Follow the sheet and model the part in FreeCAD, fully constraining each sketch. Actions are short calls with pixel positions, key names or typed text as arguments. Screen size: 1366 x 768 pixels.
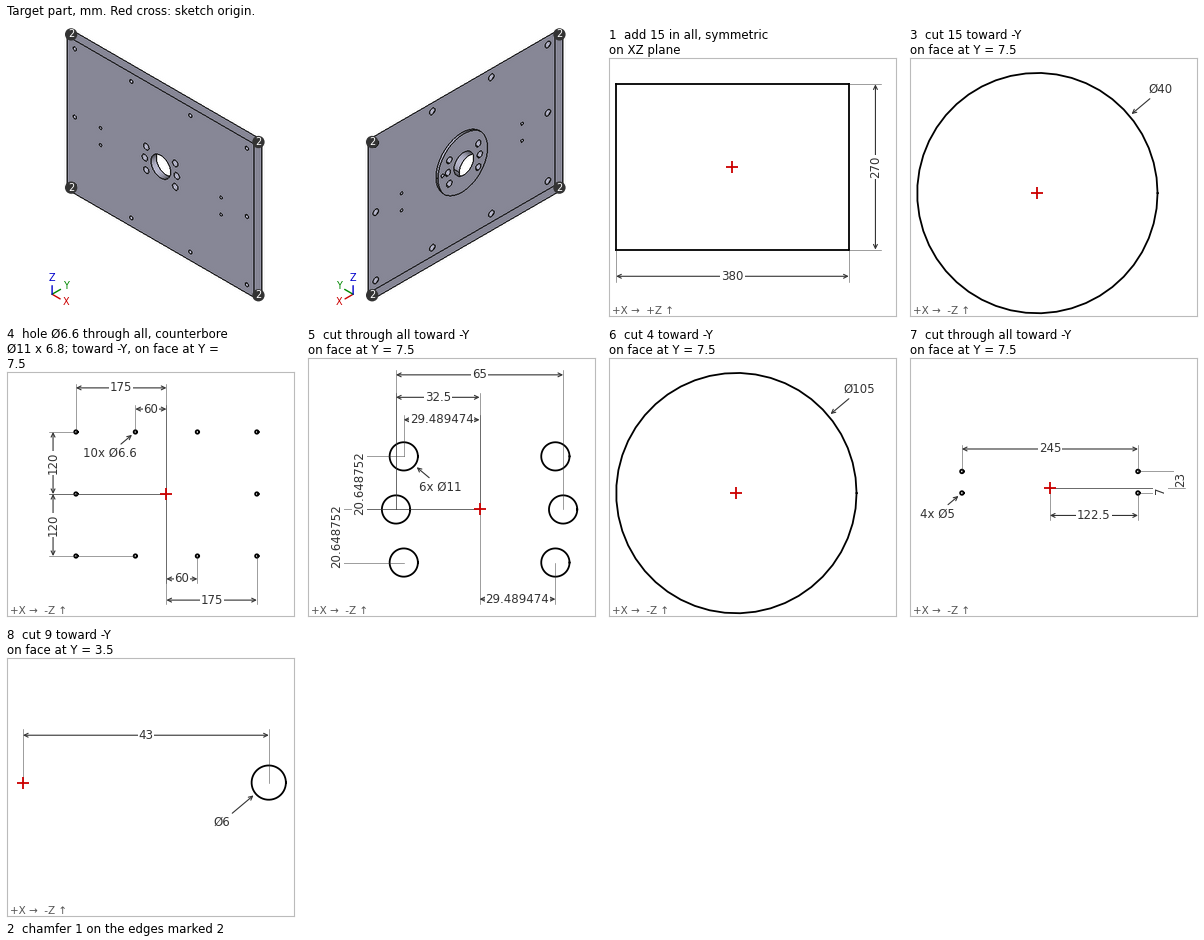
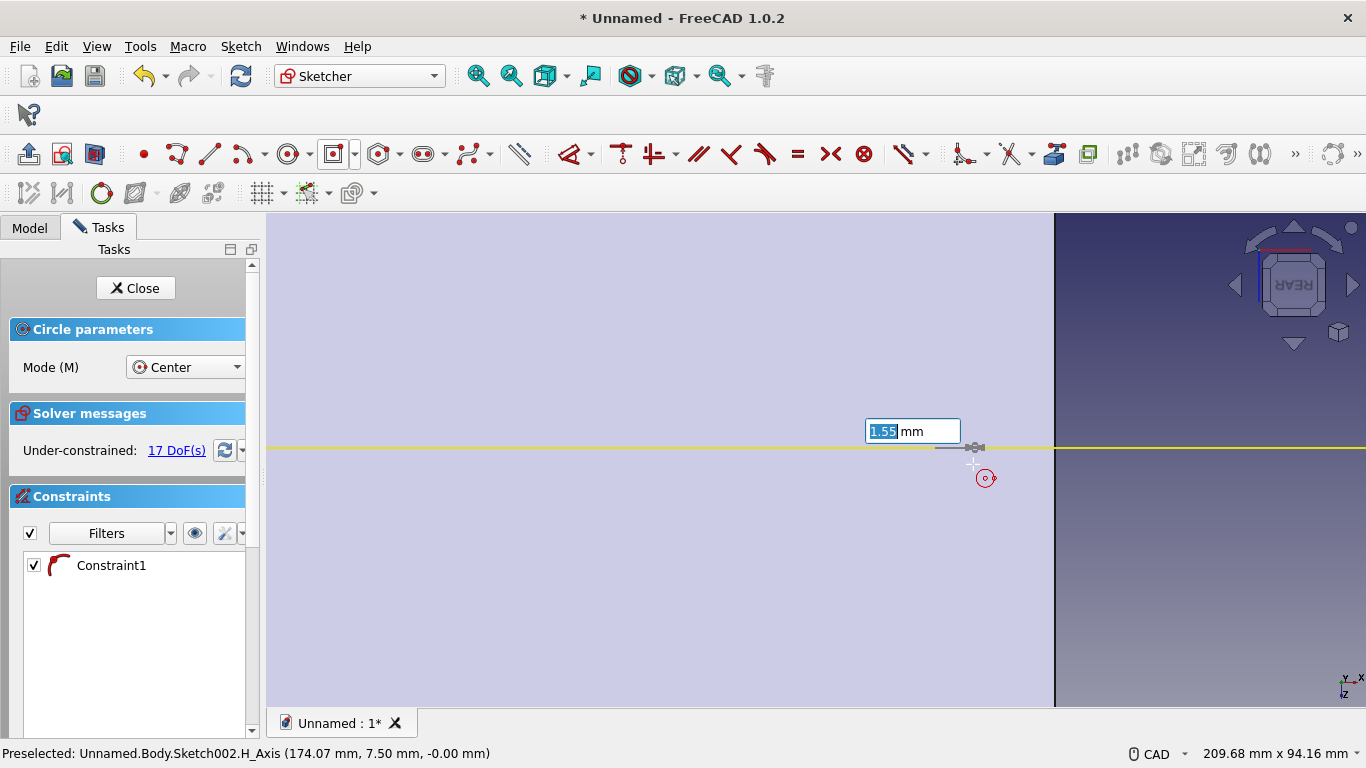
click(970, 464)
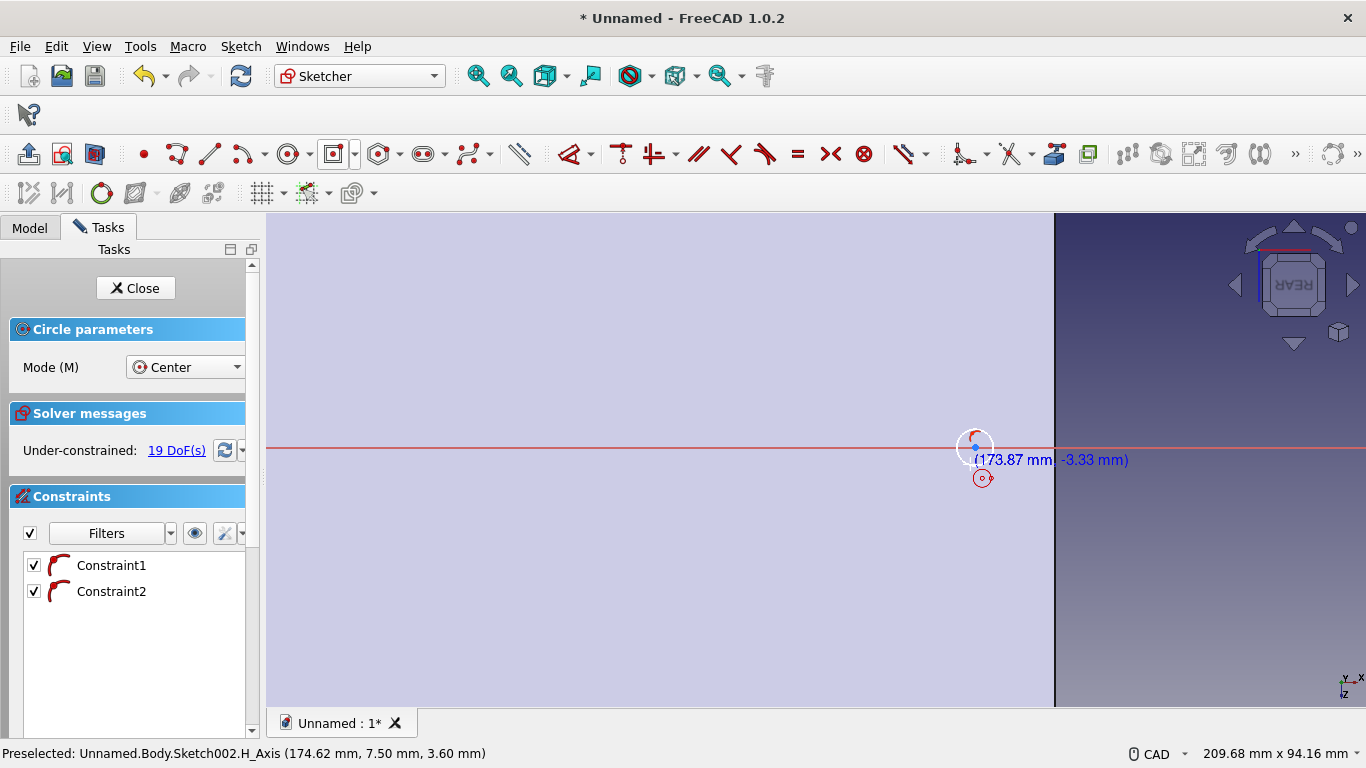
scroll(973, 464, down, 7)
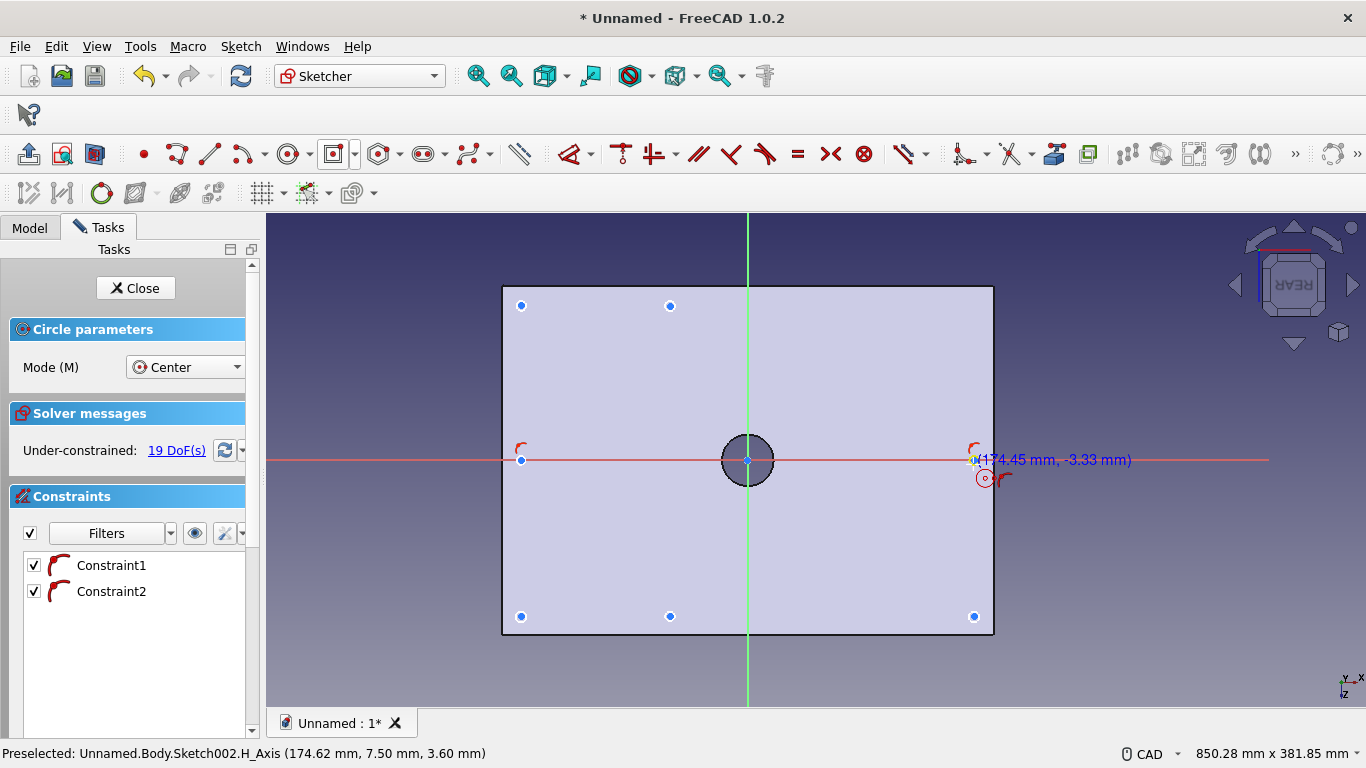
scroll(825, 616, up, 9)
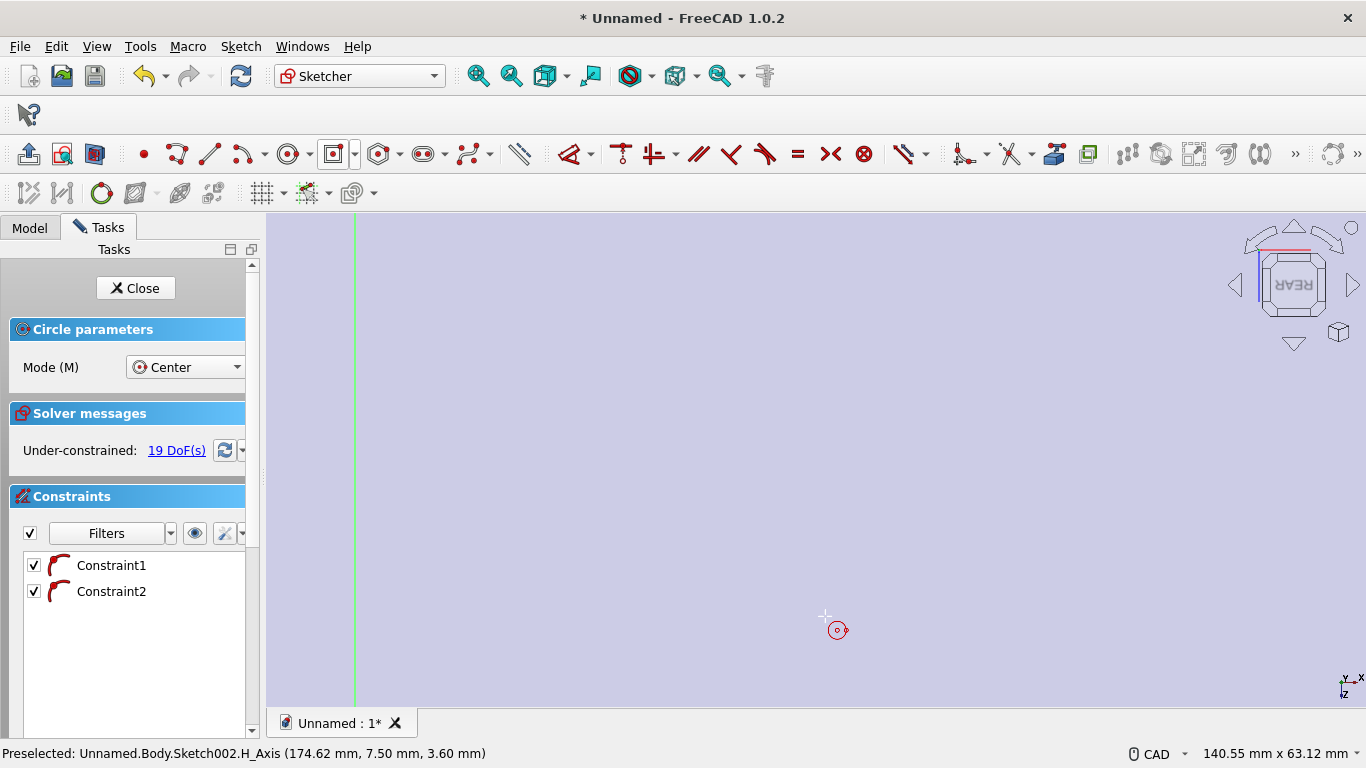
scroll(825, 616, down, 9)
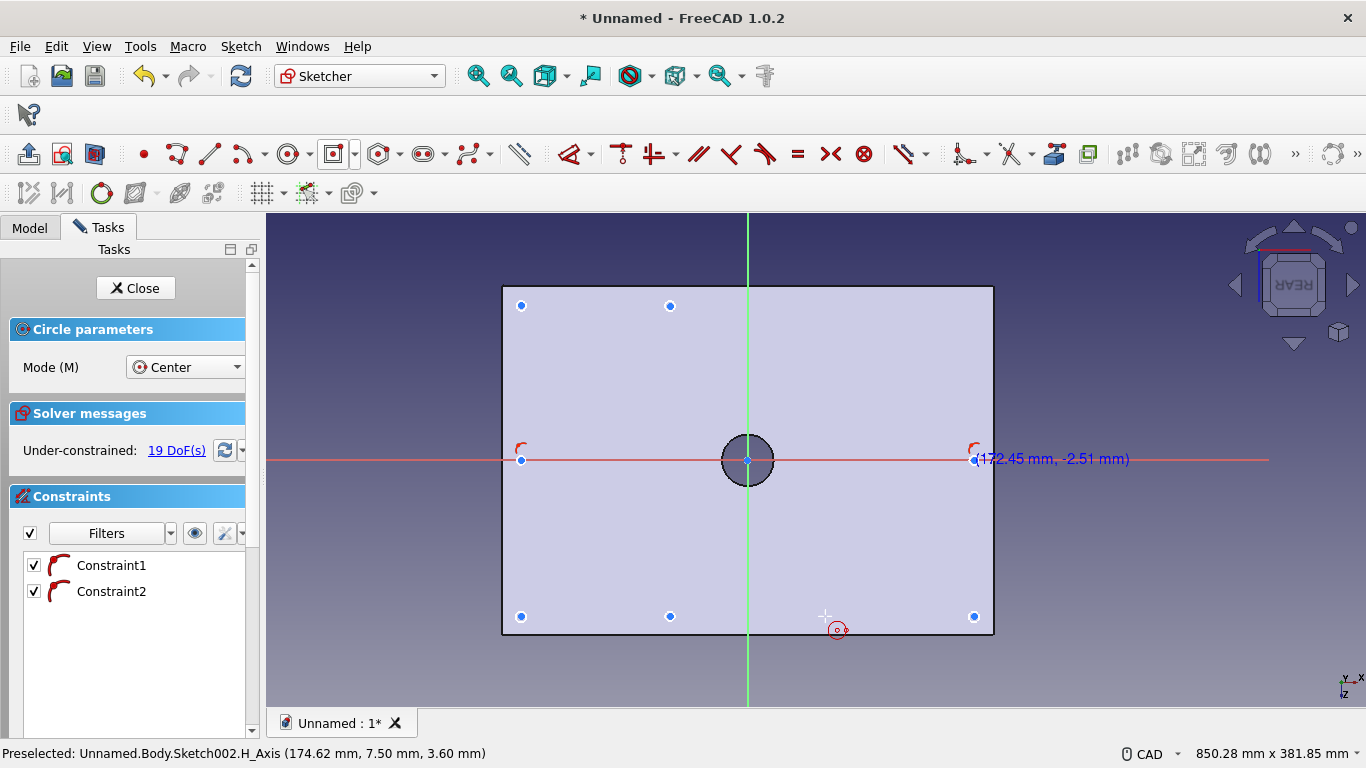
click(825, 616)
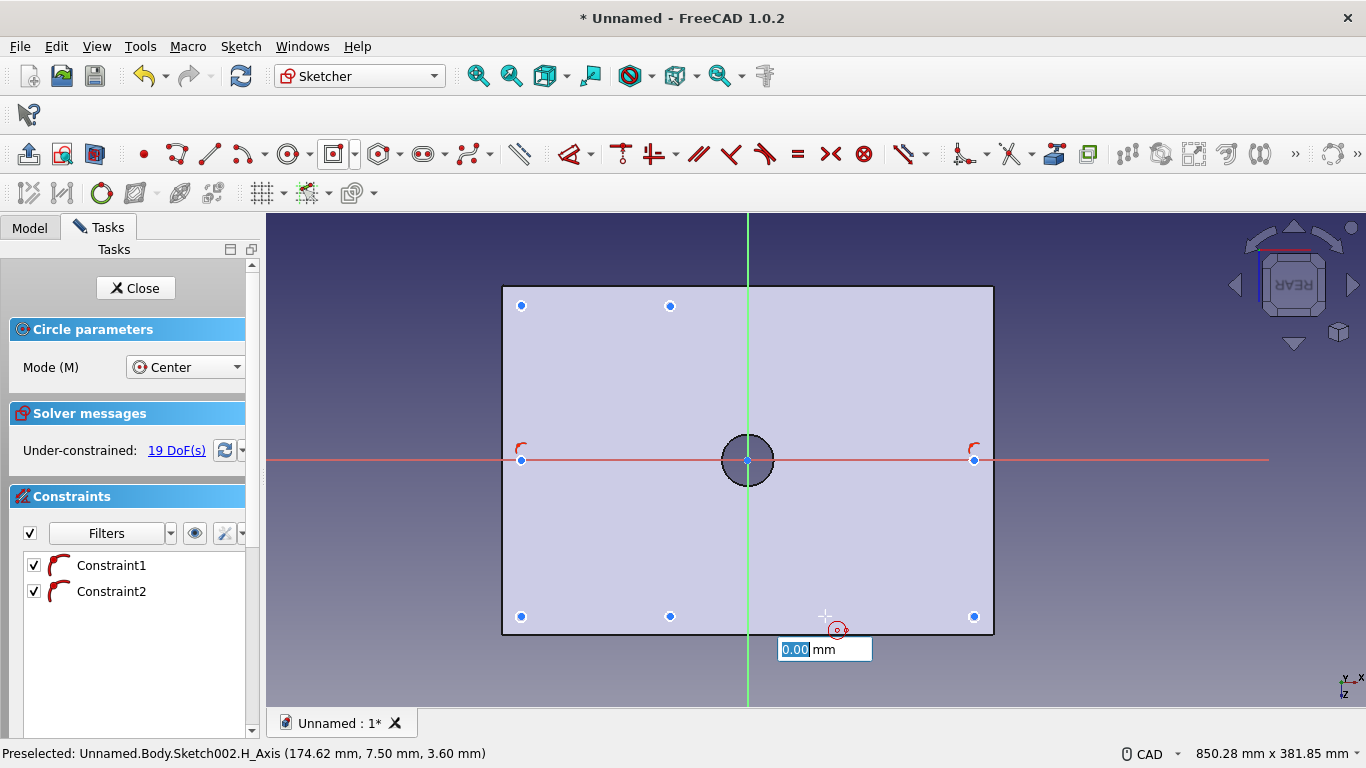
scroll(828, 613, up, 7)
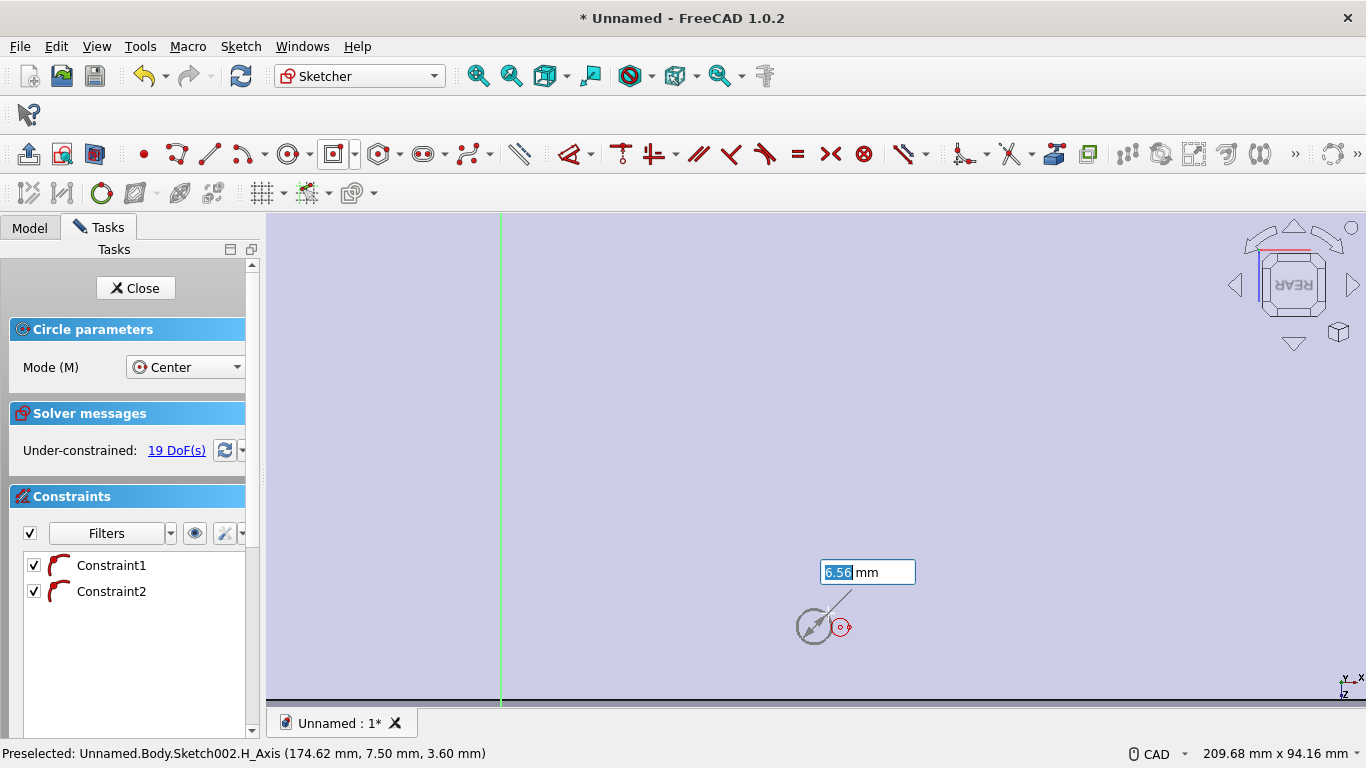
click(828, 609)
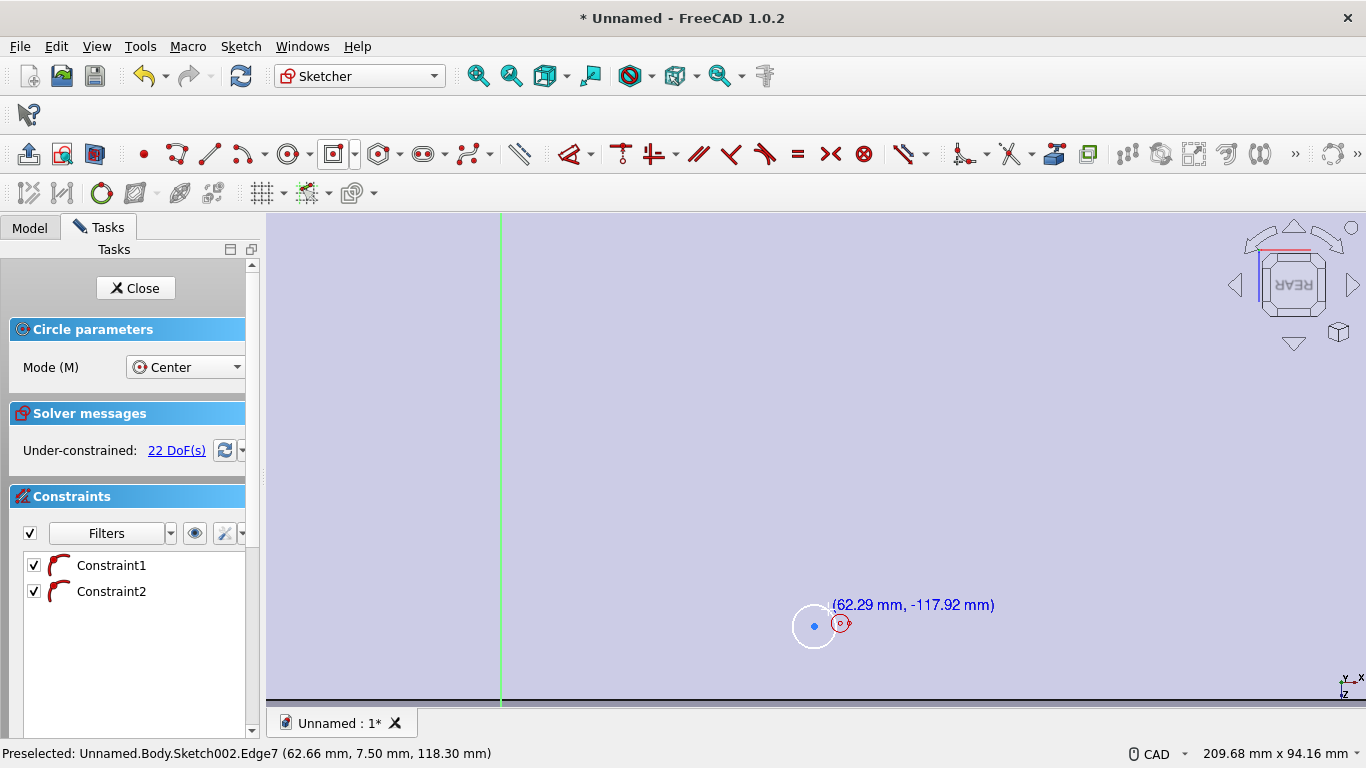
scroll(828, 613, down, 7)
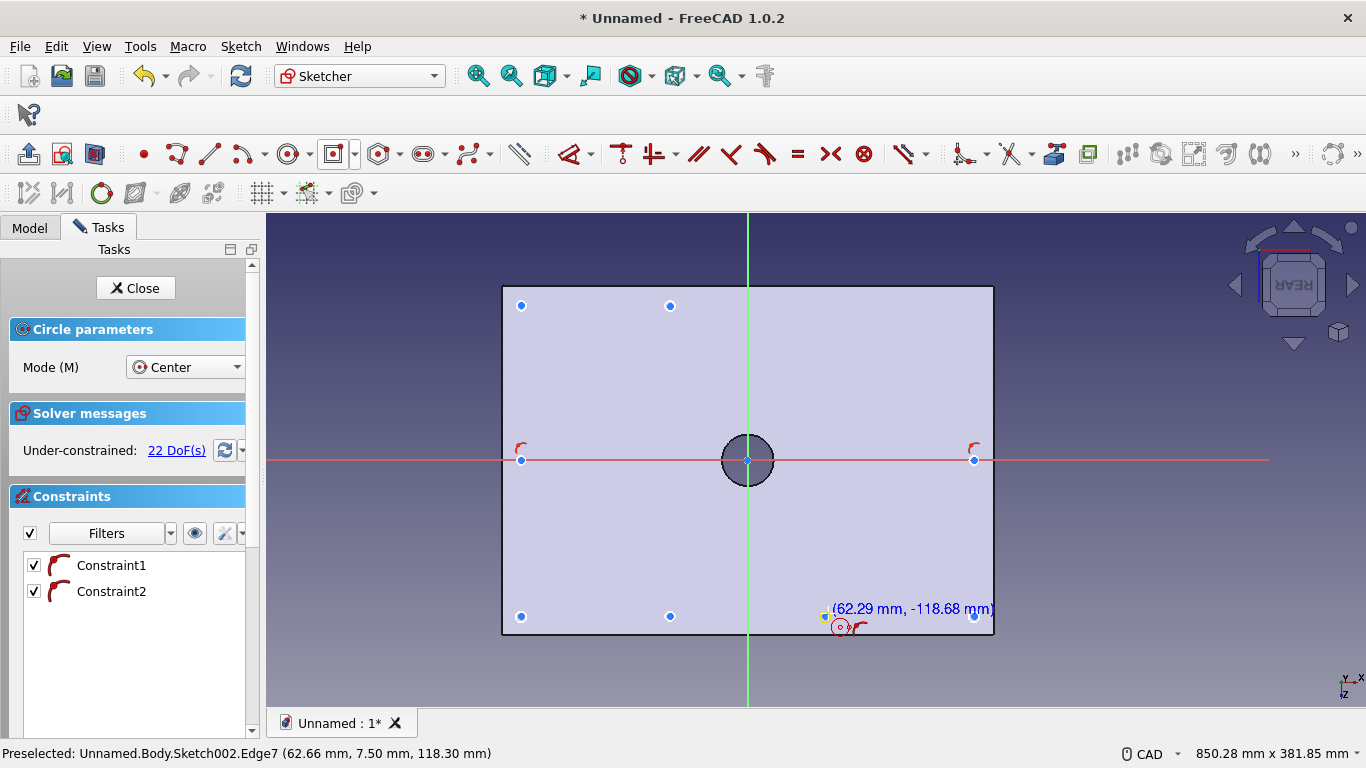
scroll(825, 305, up, 9)